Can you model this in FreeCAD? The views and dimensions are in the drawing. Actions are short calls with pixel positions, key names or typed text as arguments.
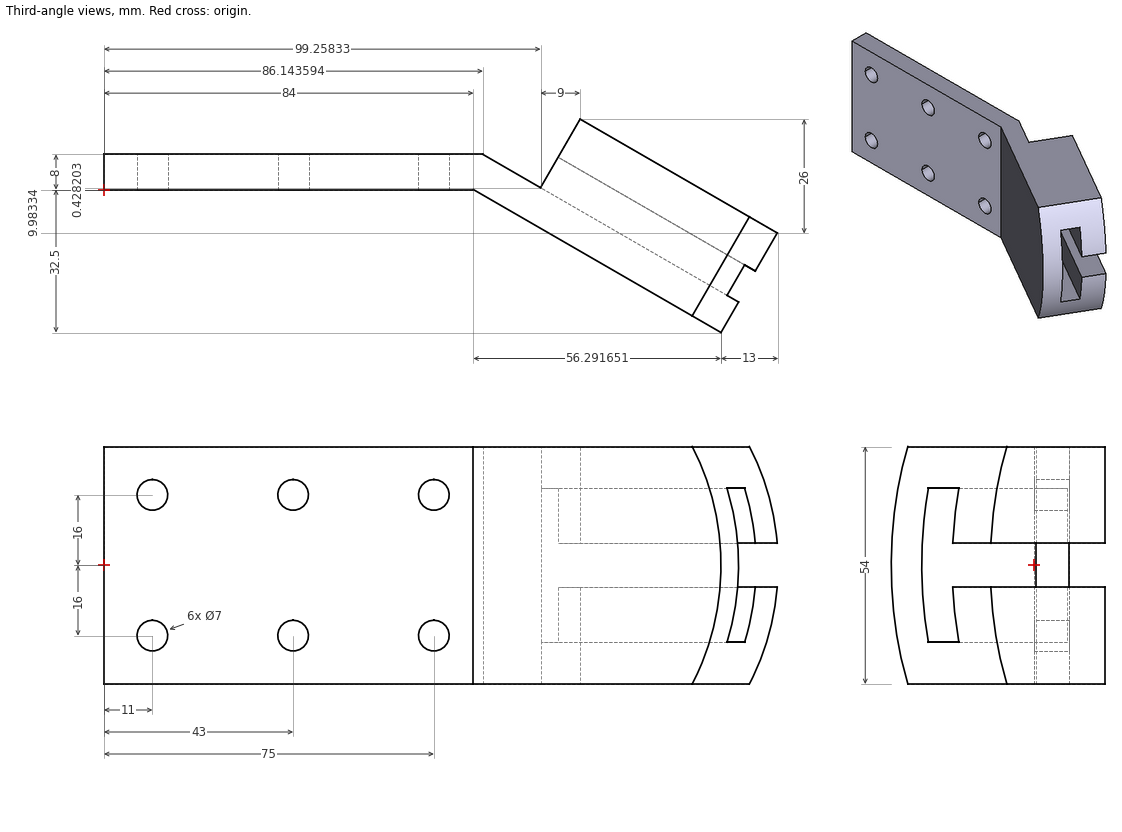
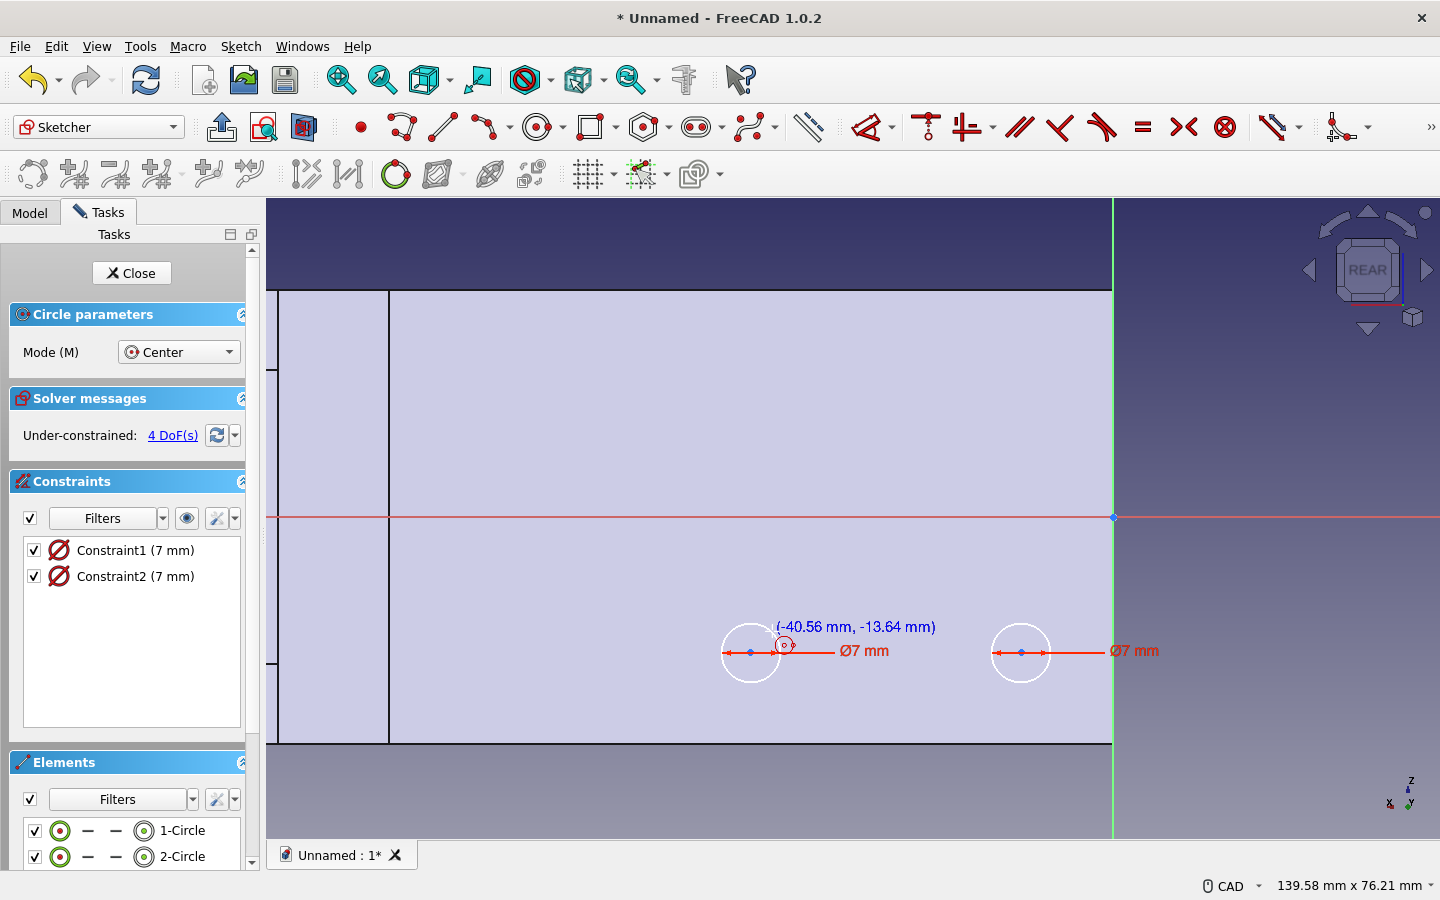
click(482, 652)
move(503, 631)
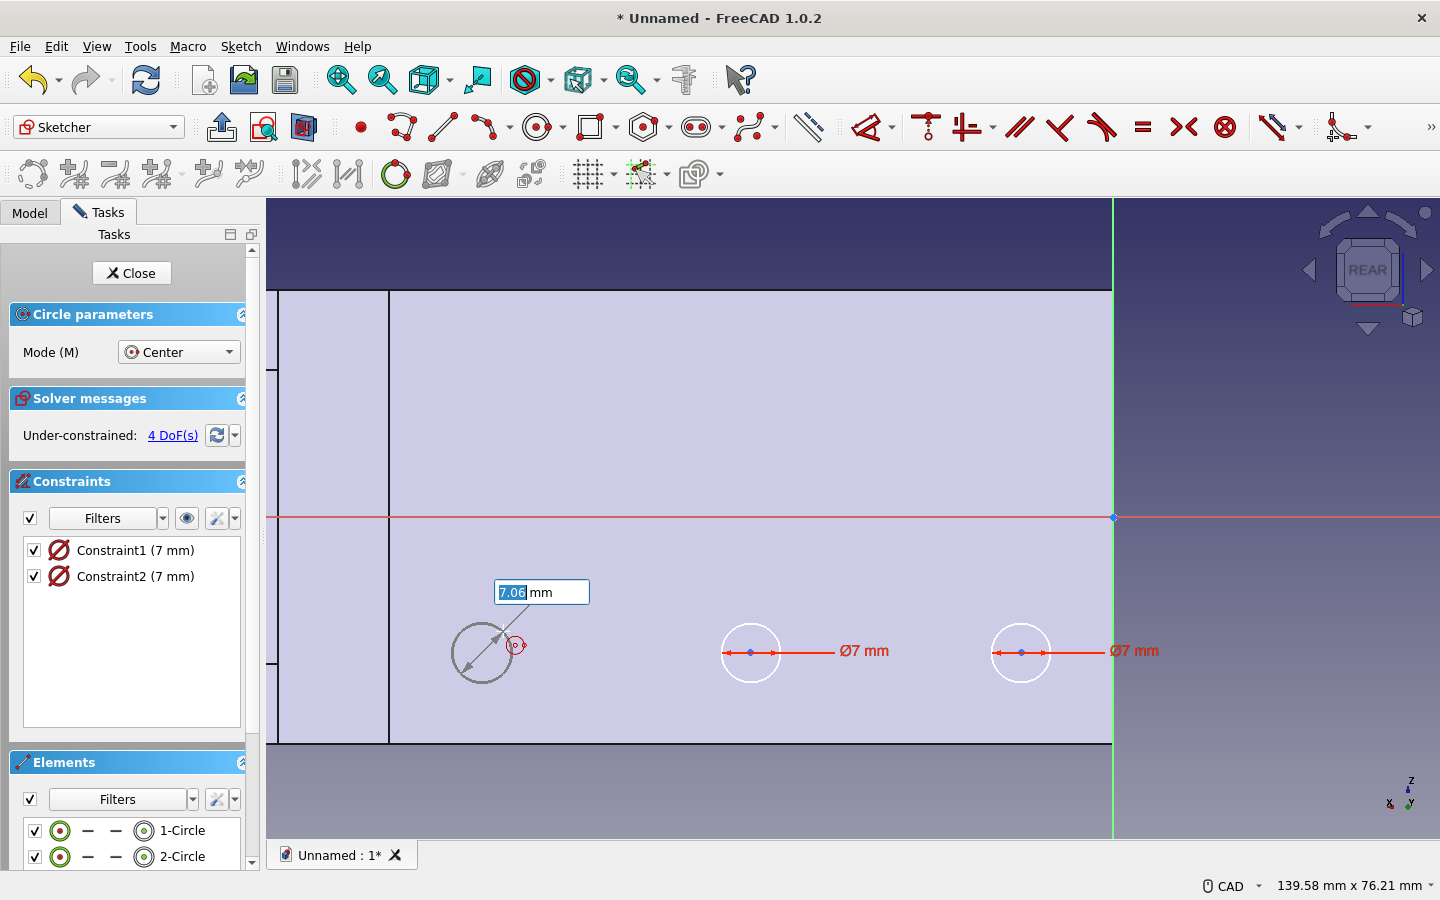
text(7)
key(Return)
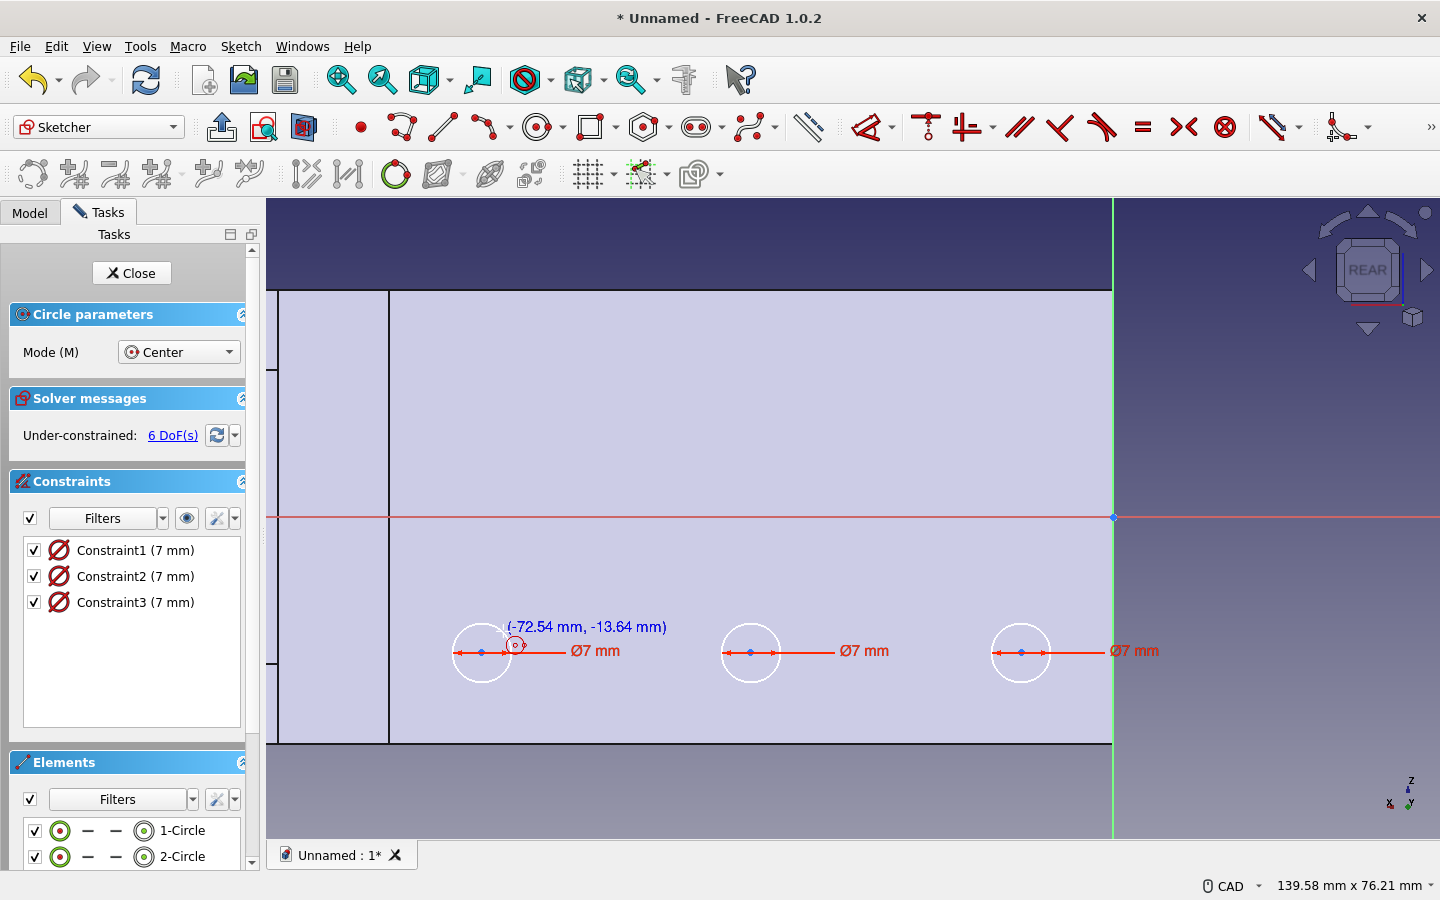
click(1021, 383)
move(1041, 362)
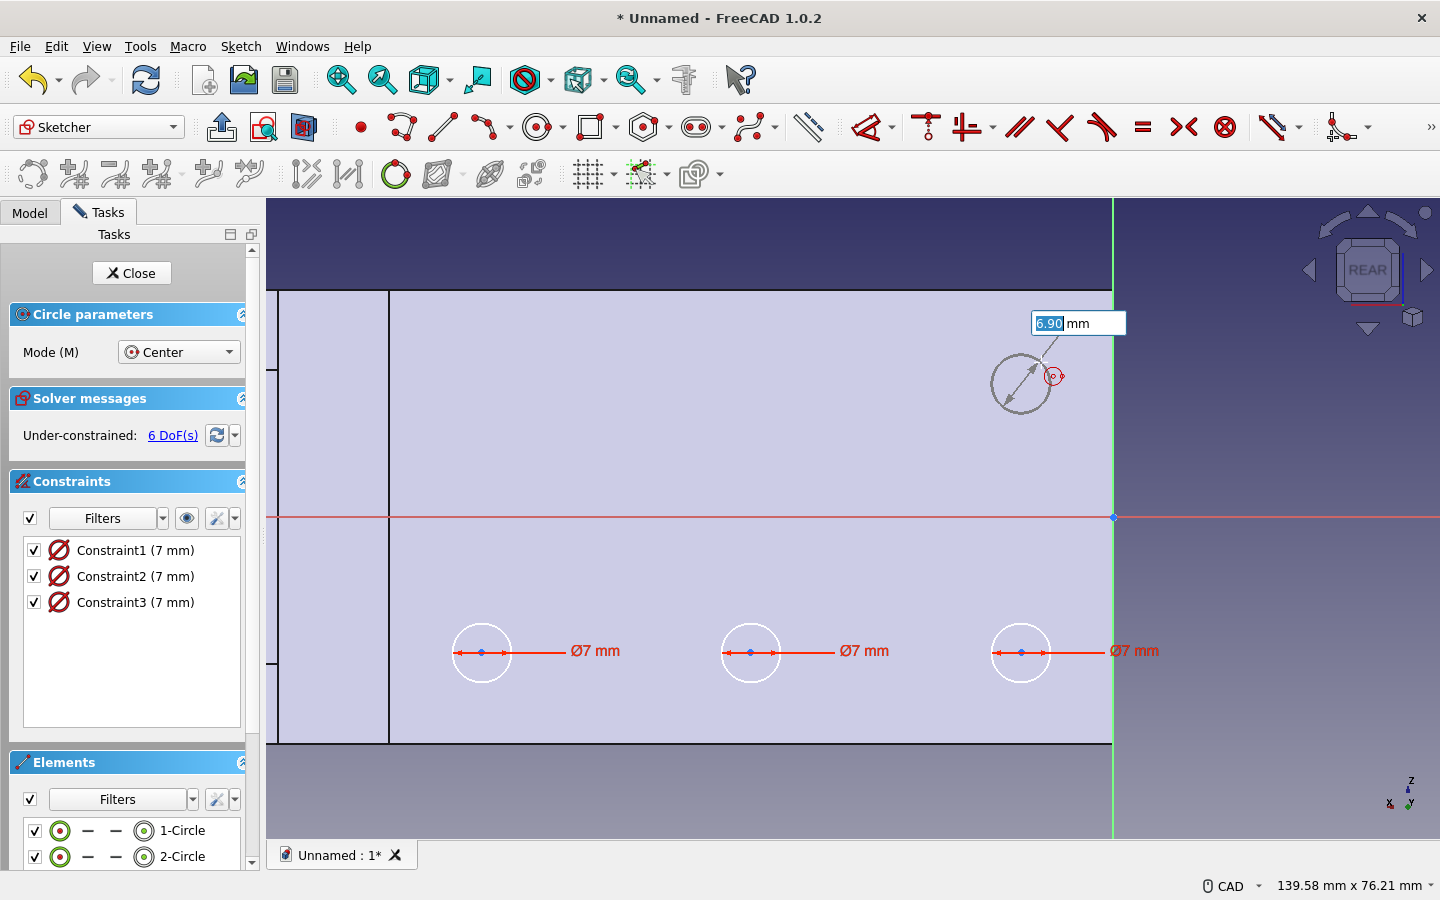
text(7)
key(Return)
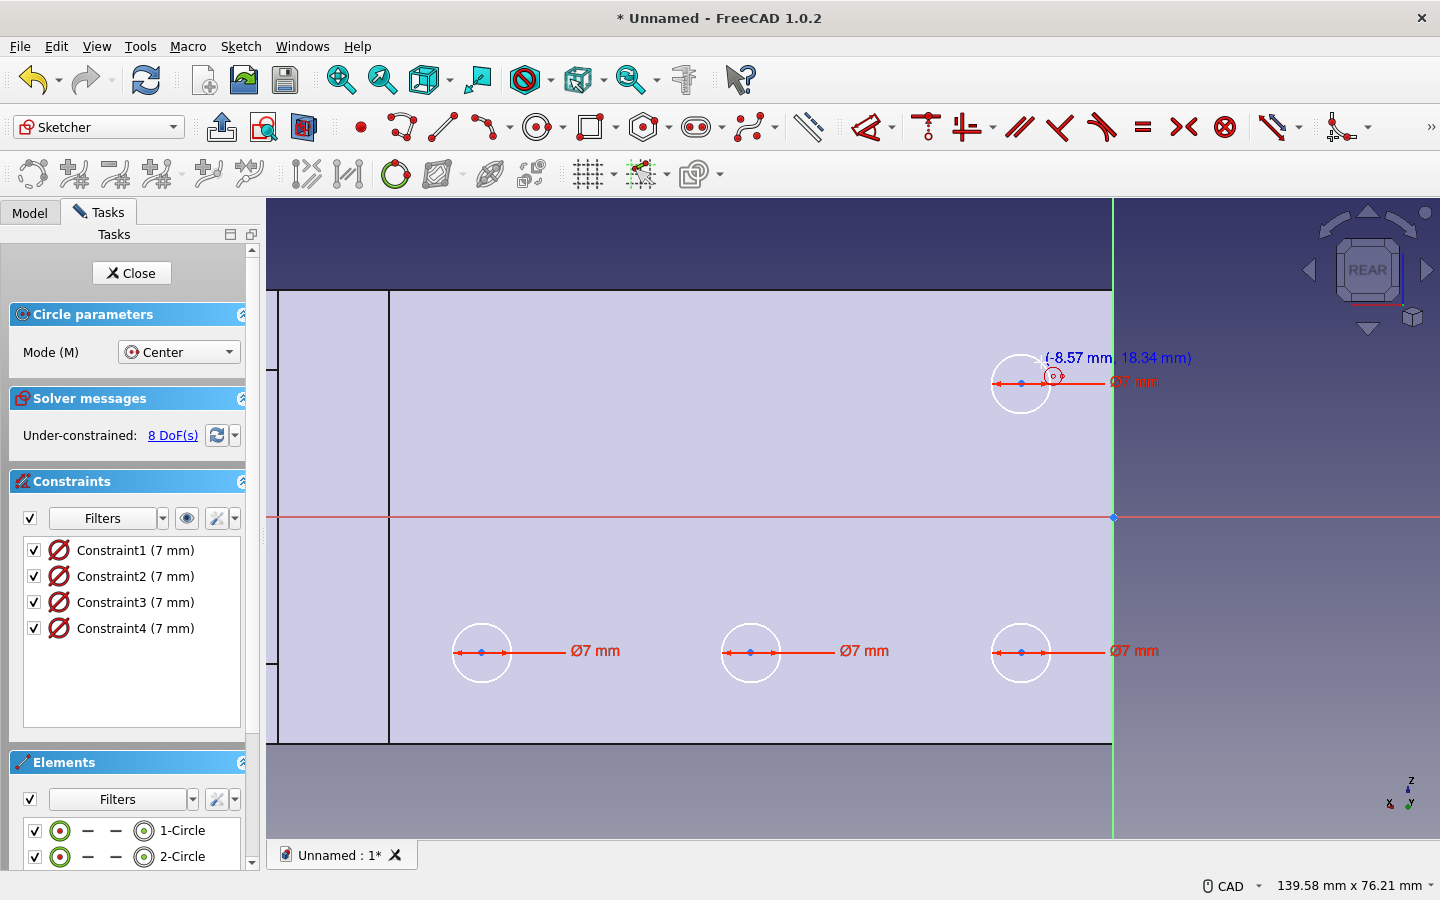
click(751, 383)
move(772, 362)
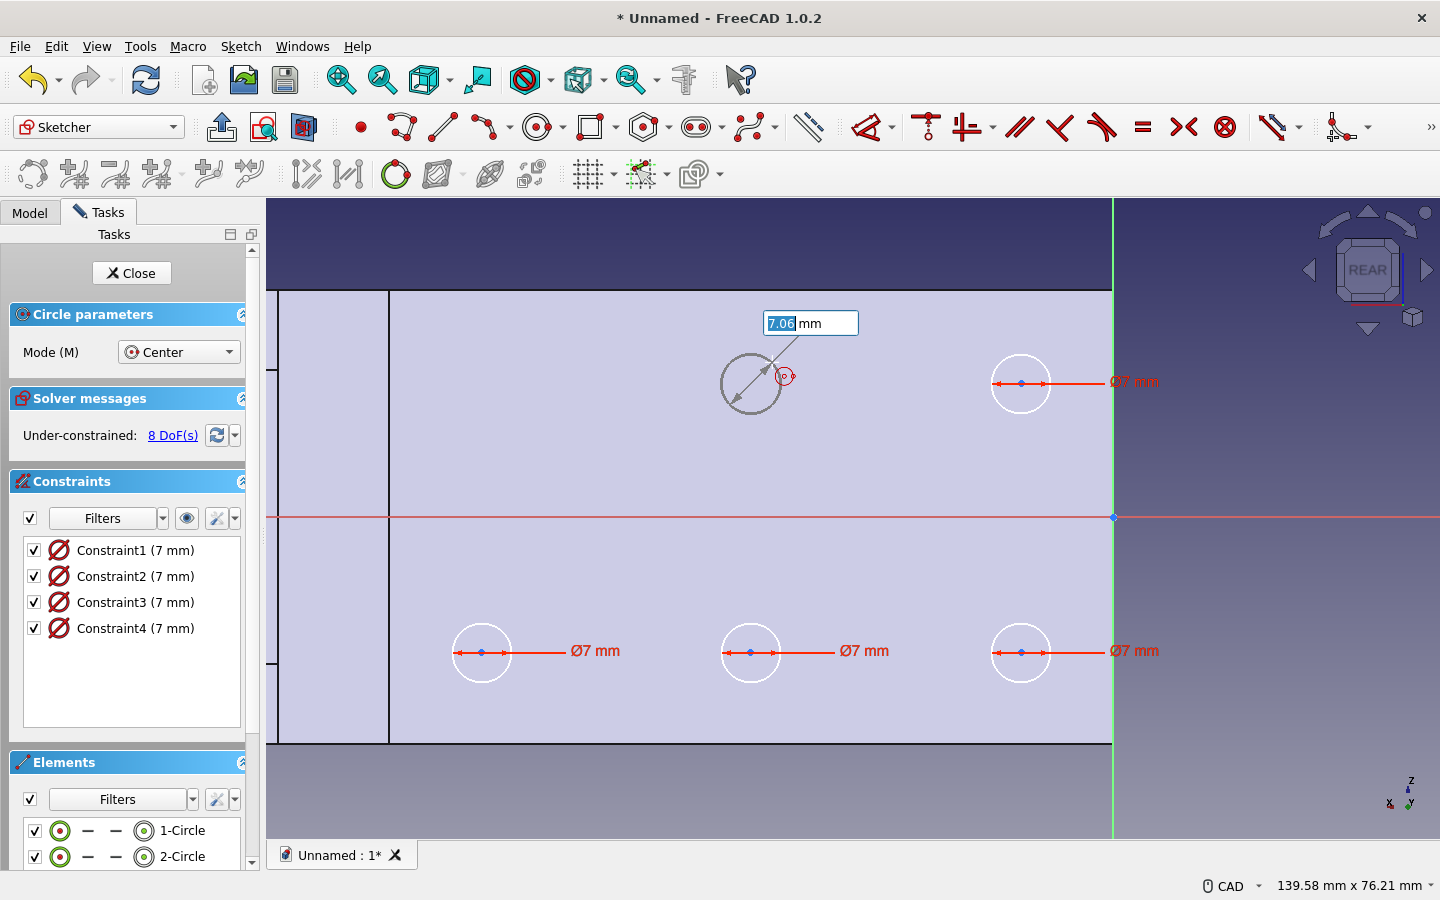
text(7)
key(Return)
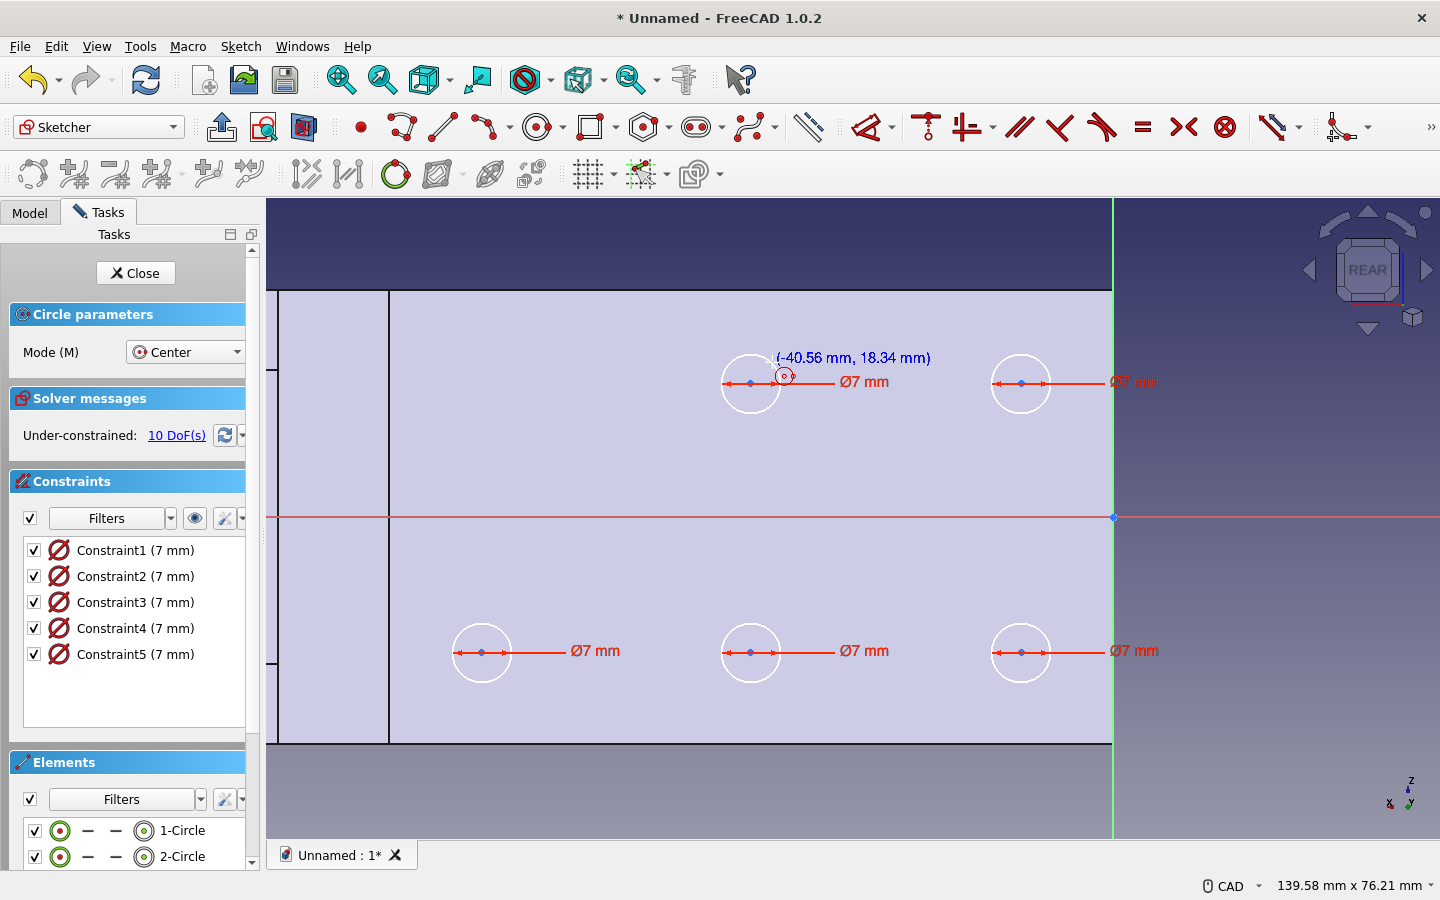
click(482, 383)
move(503, 362)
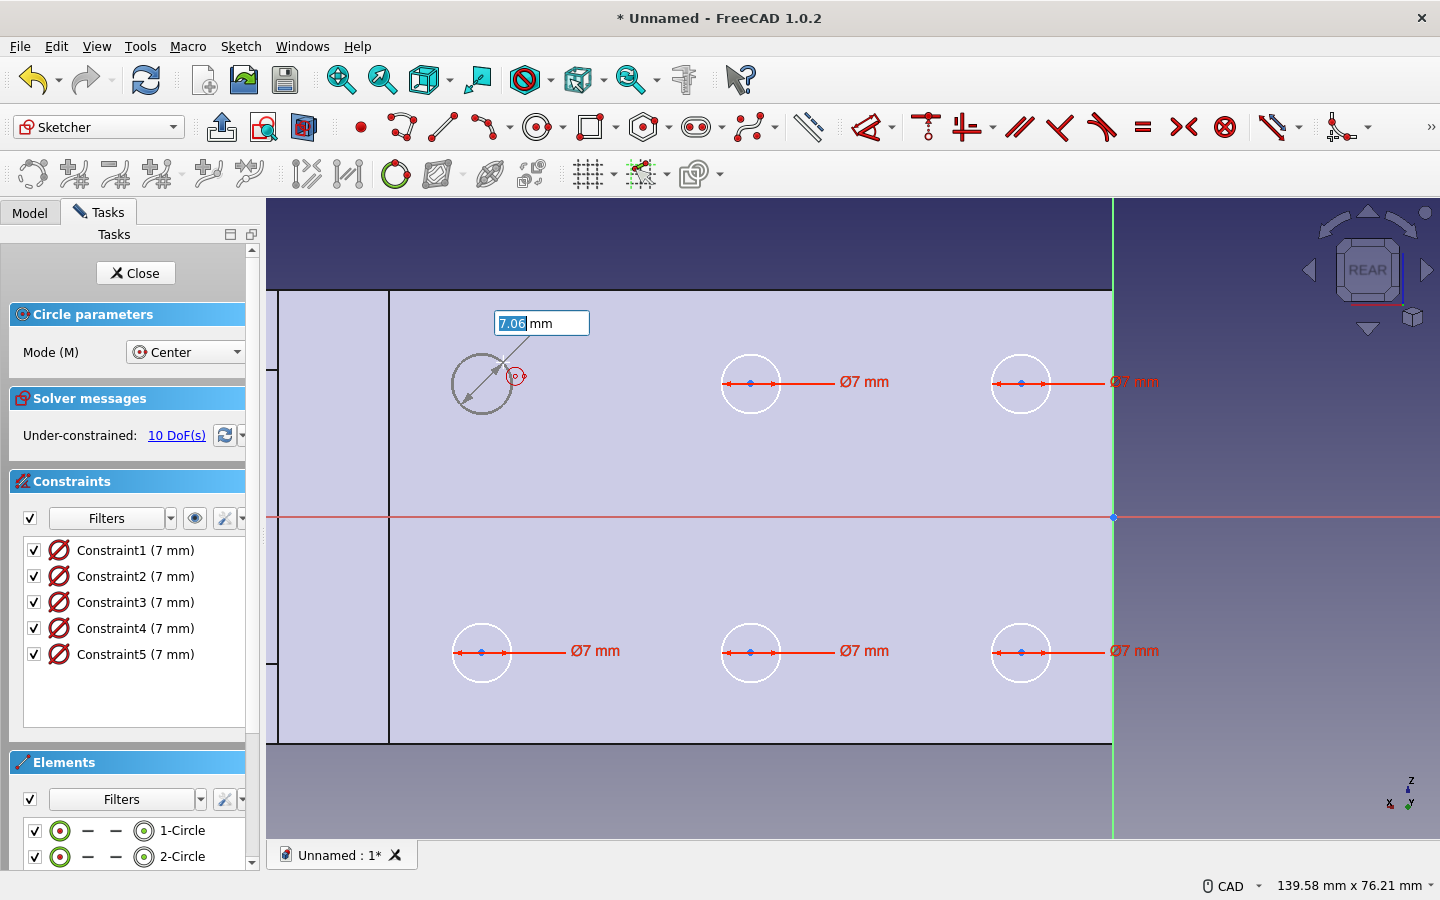
text(7)
key(Return)
key(Escape)